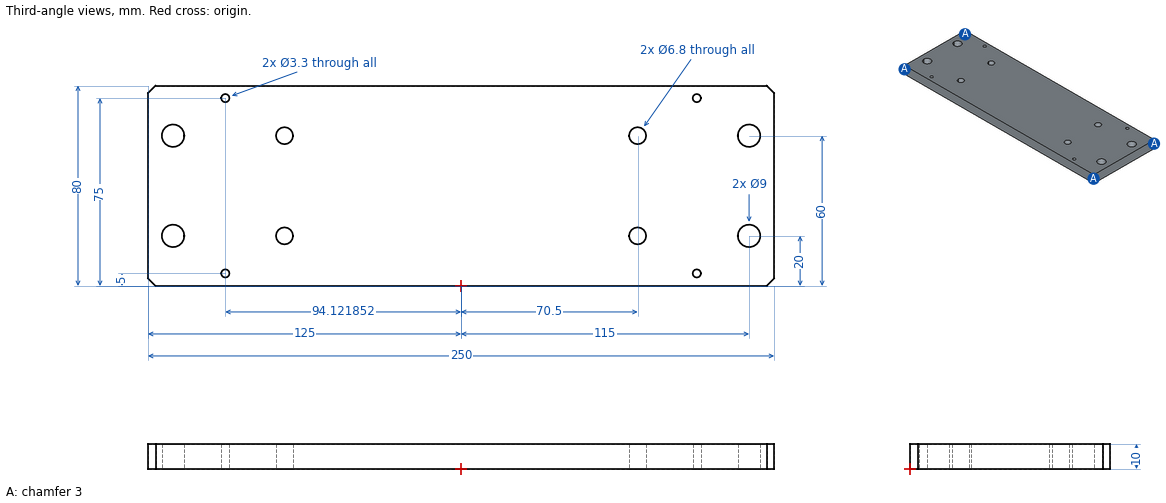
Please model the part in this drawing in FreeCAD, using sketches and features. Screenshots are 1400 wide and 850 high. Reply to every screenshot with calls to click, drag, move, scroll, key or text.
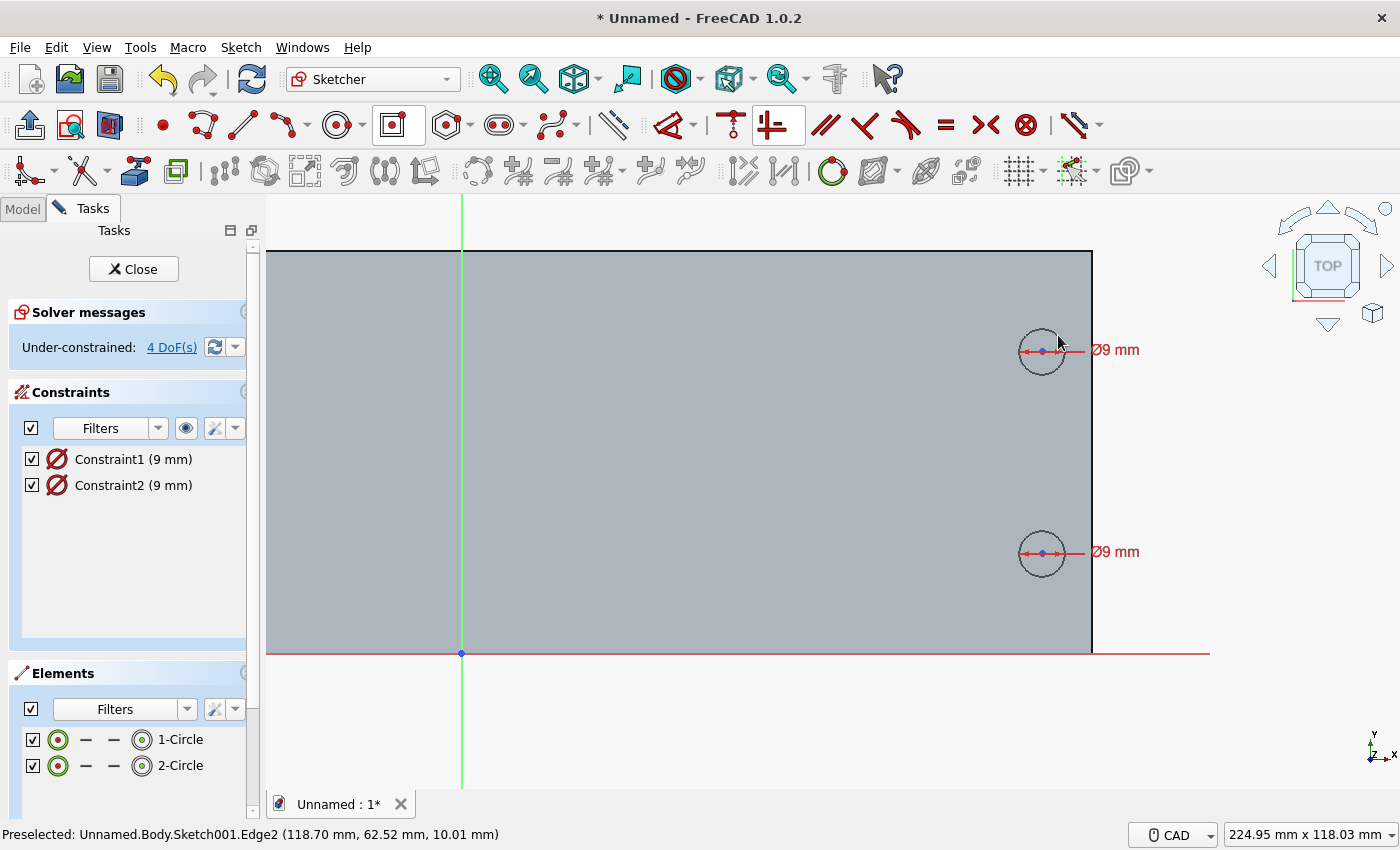
click(1042, 554)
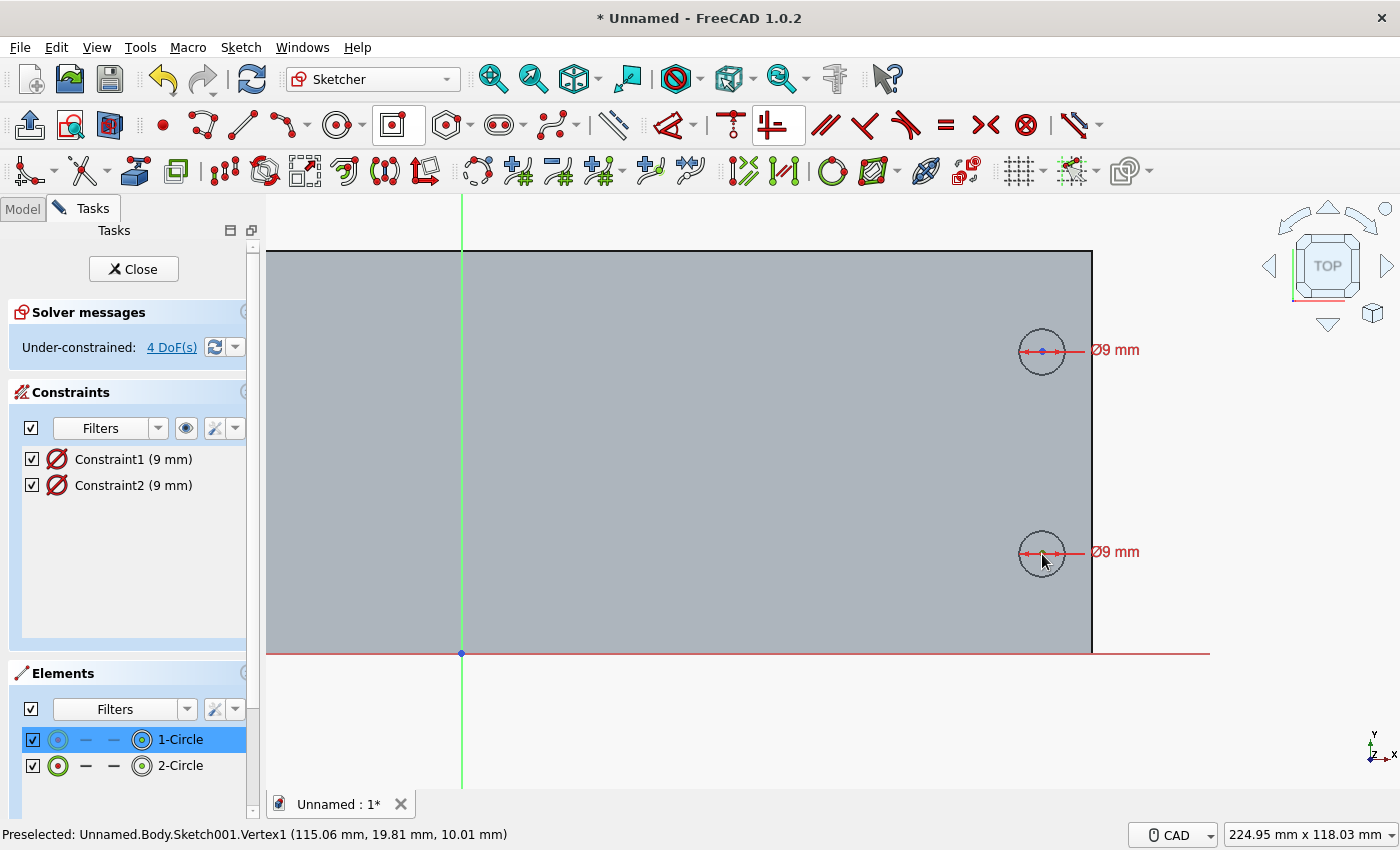
click(1042, 352)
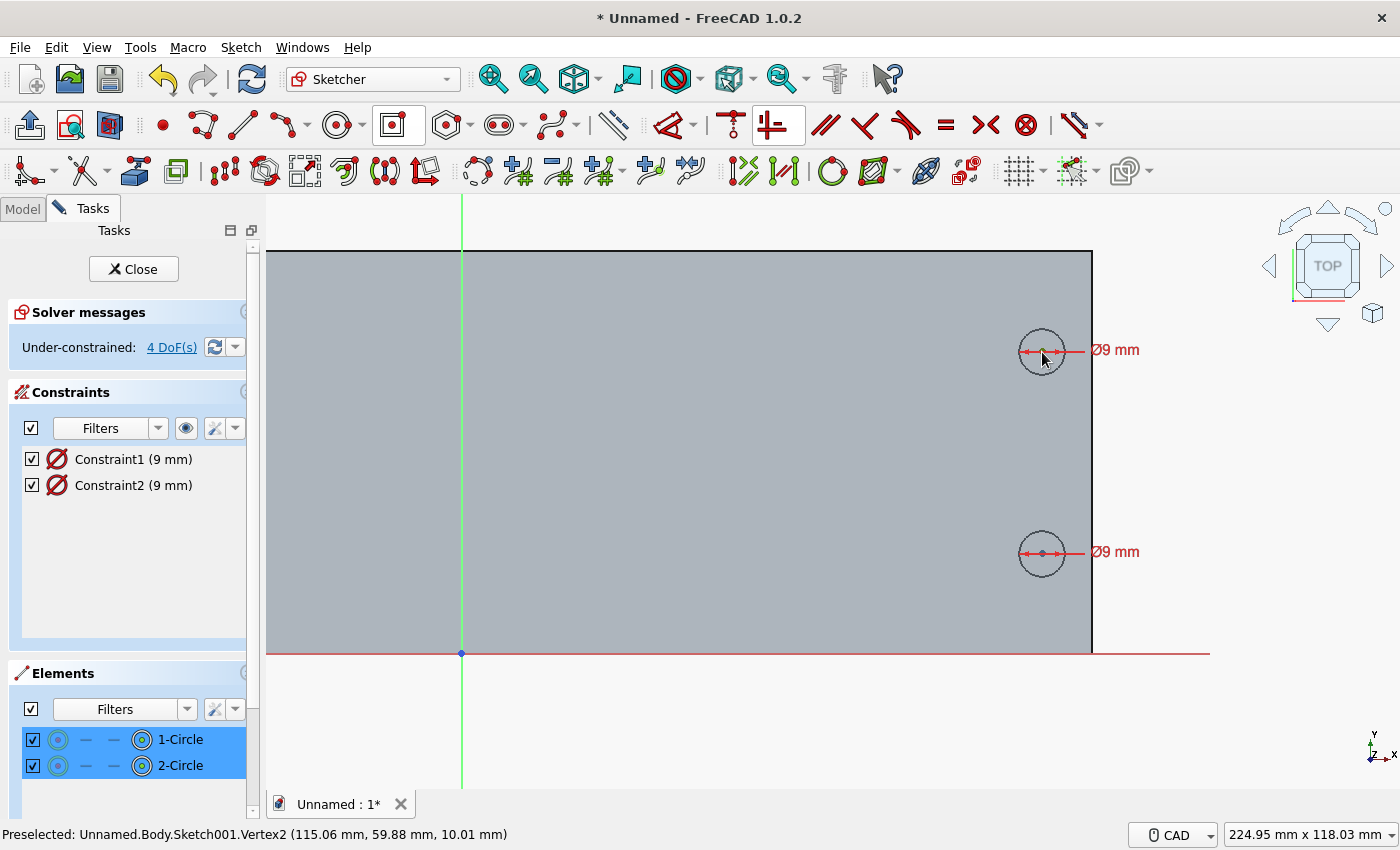
click(800, 126)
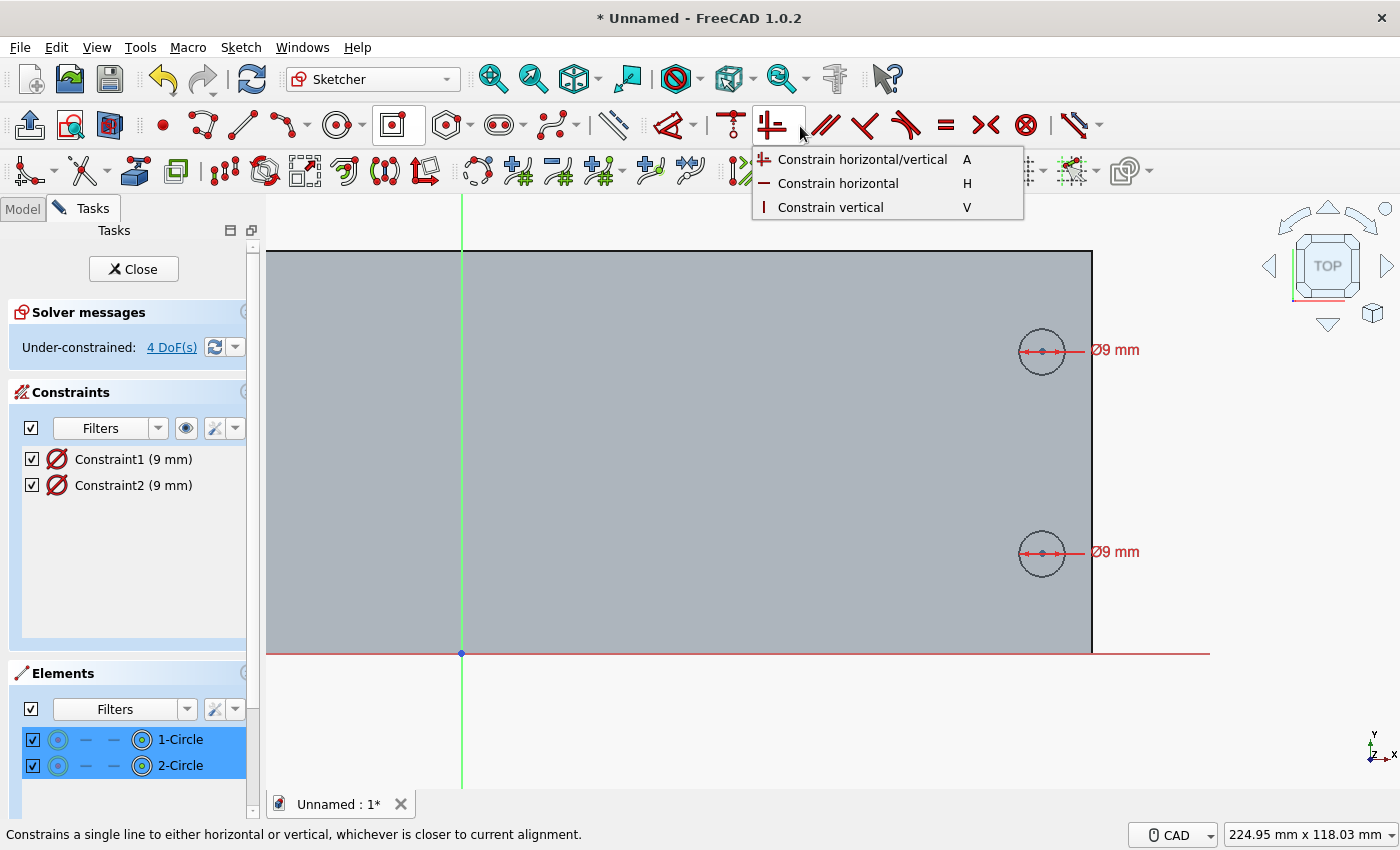
click(888, 207)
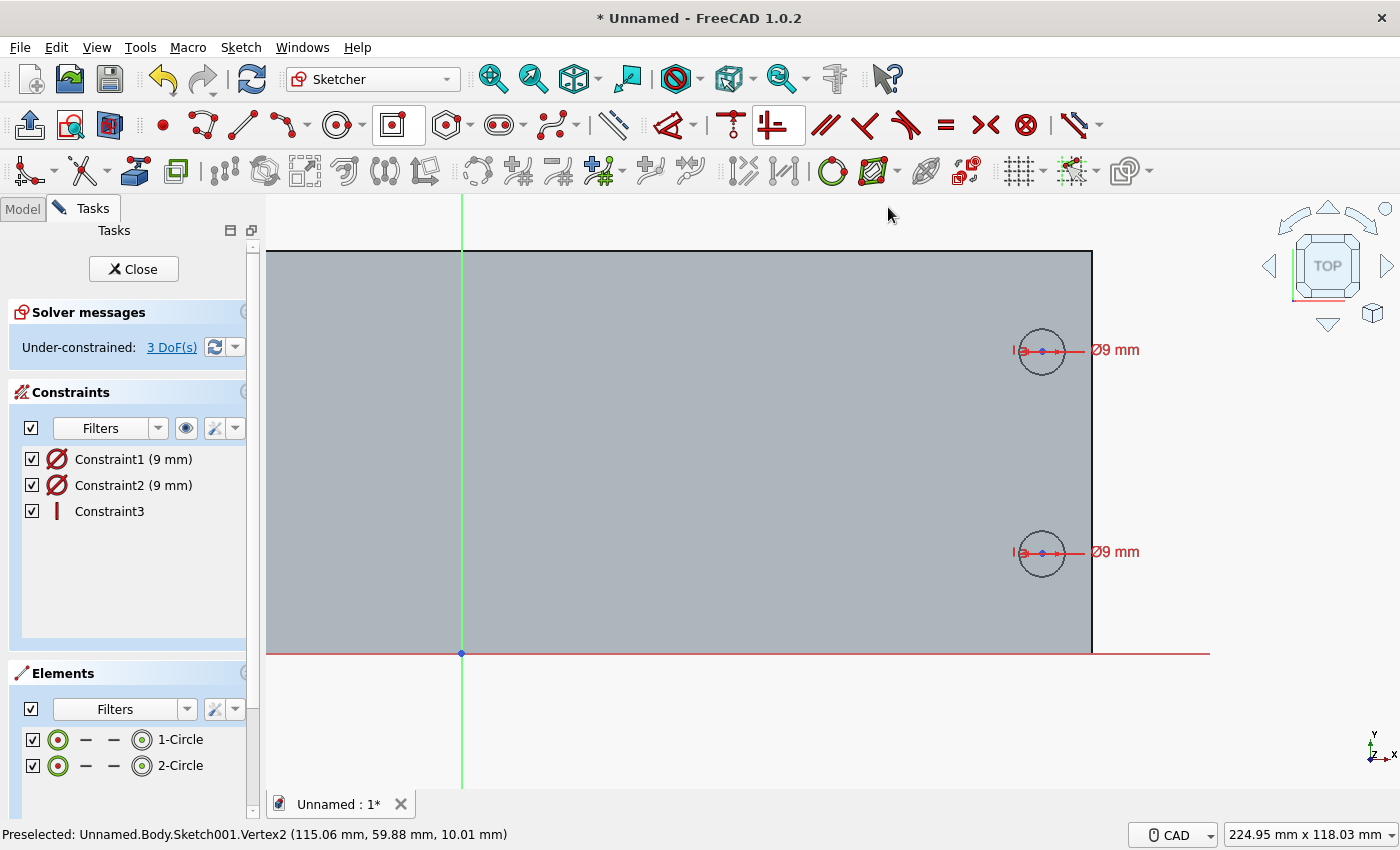
click(668, 126)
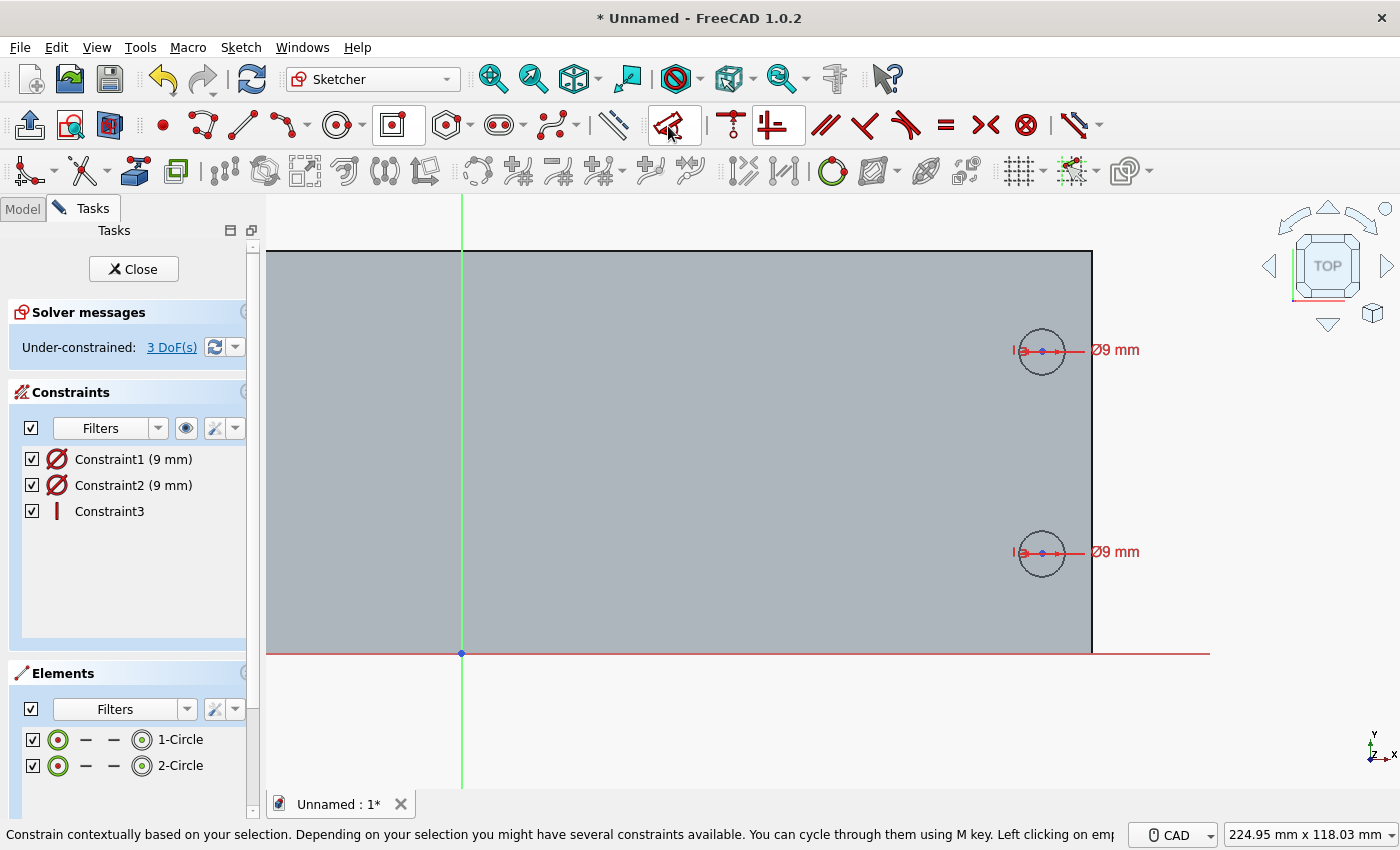
click(1042, 554)
click(428, 604)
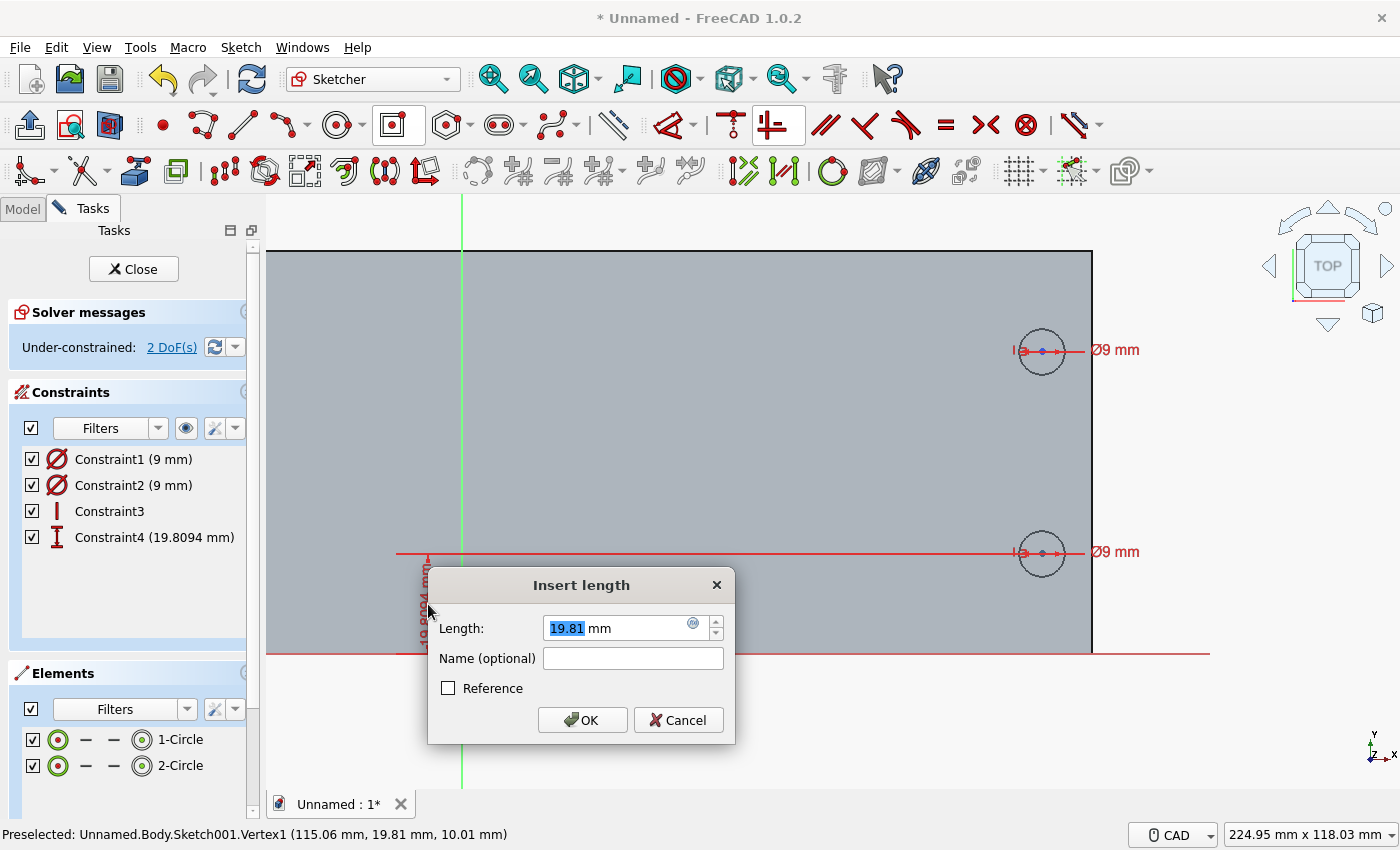
text(20)
key(Return)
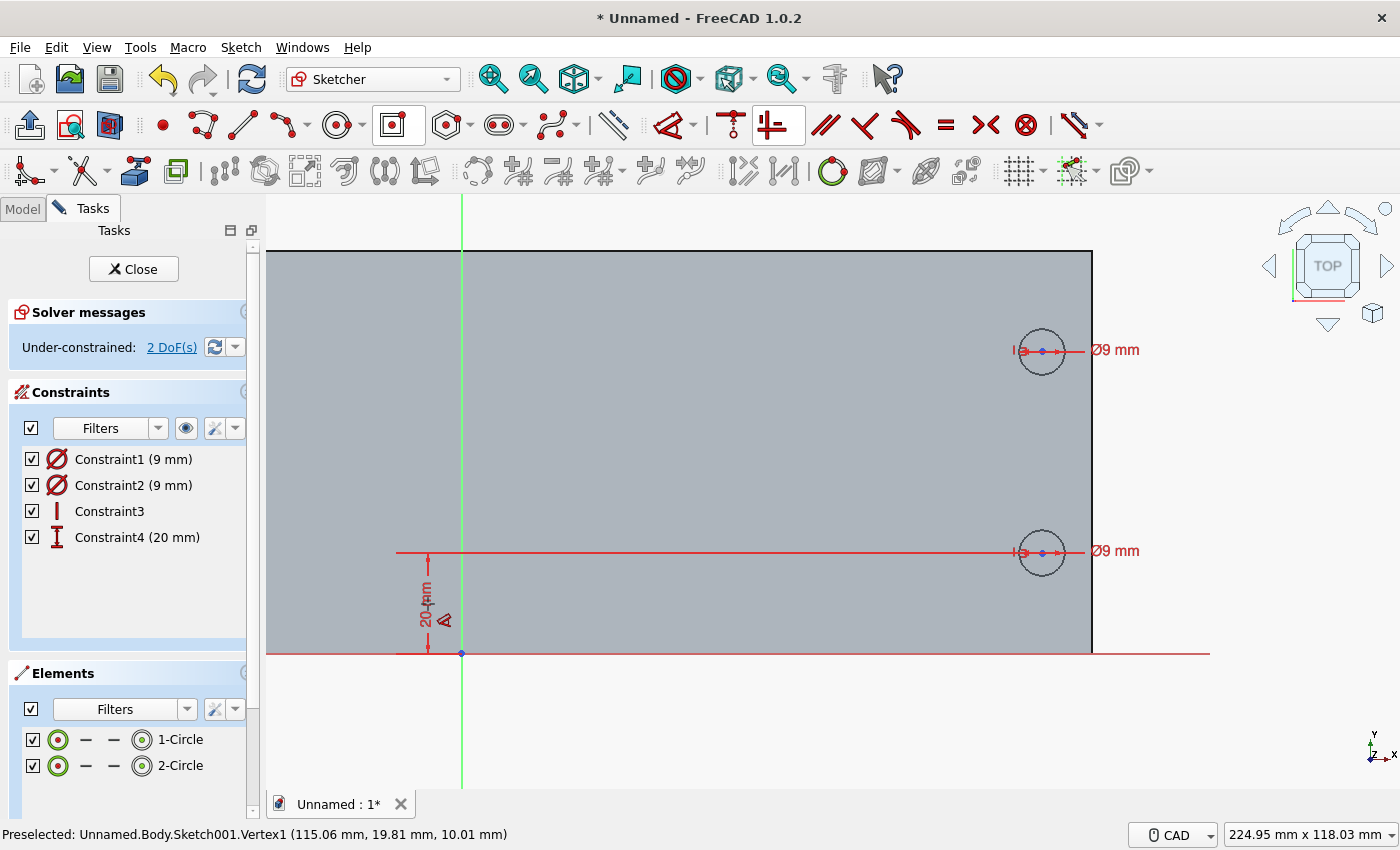
click(1042, 352)
click(428, 503)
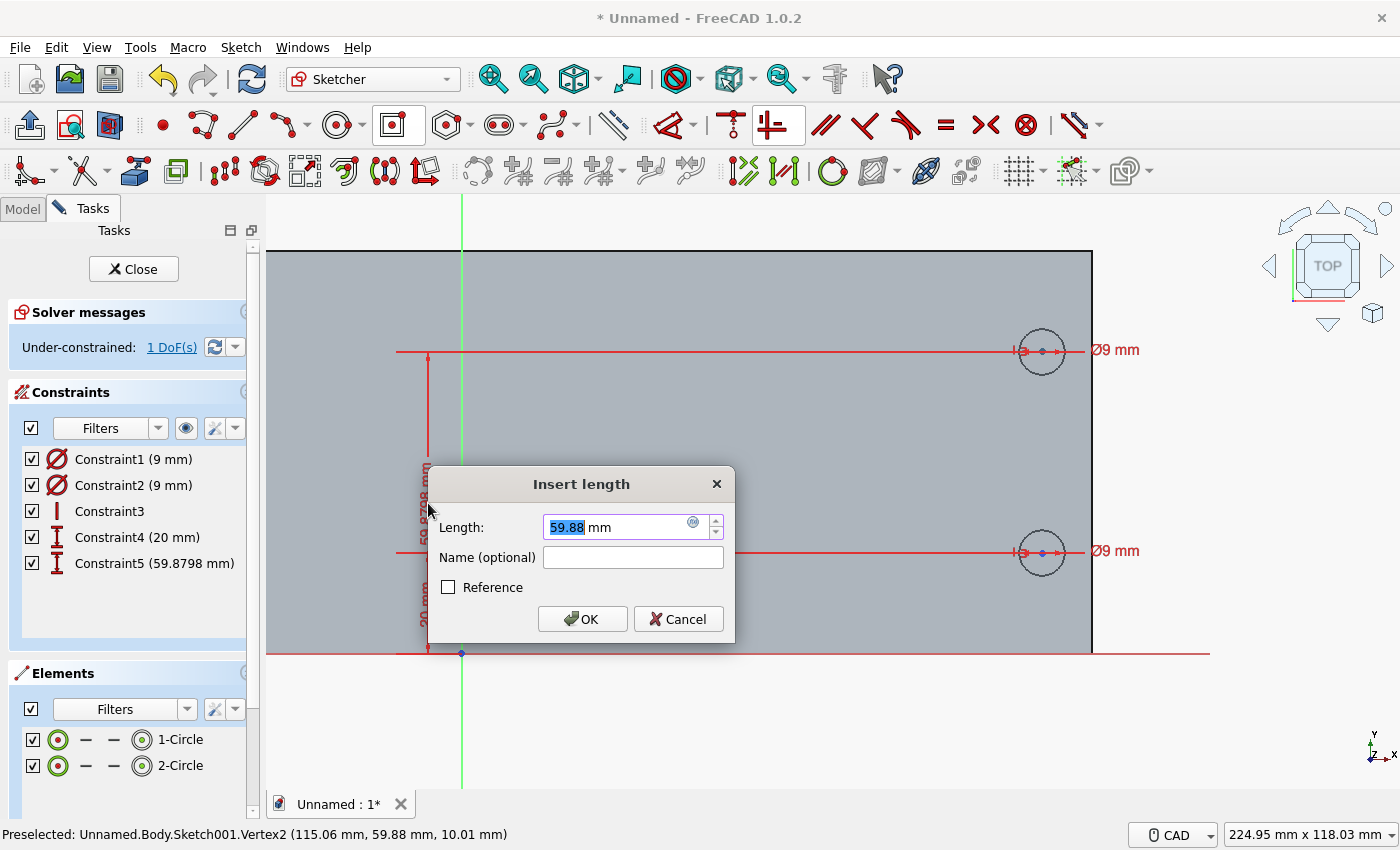
text(60)
key(Return)